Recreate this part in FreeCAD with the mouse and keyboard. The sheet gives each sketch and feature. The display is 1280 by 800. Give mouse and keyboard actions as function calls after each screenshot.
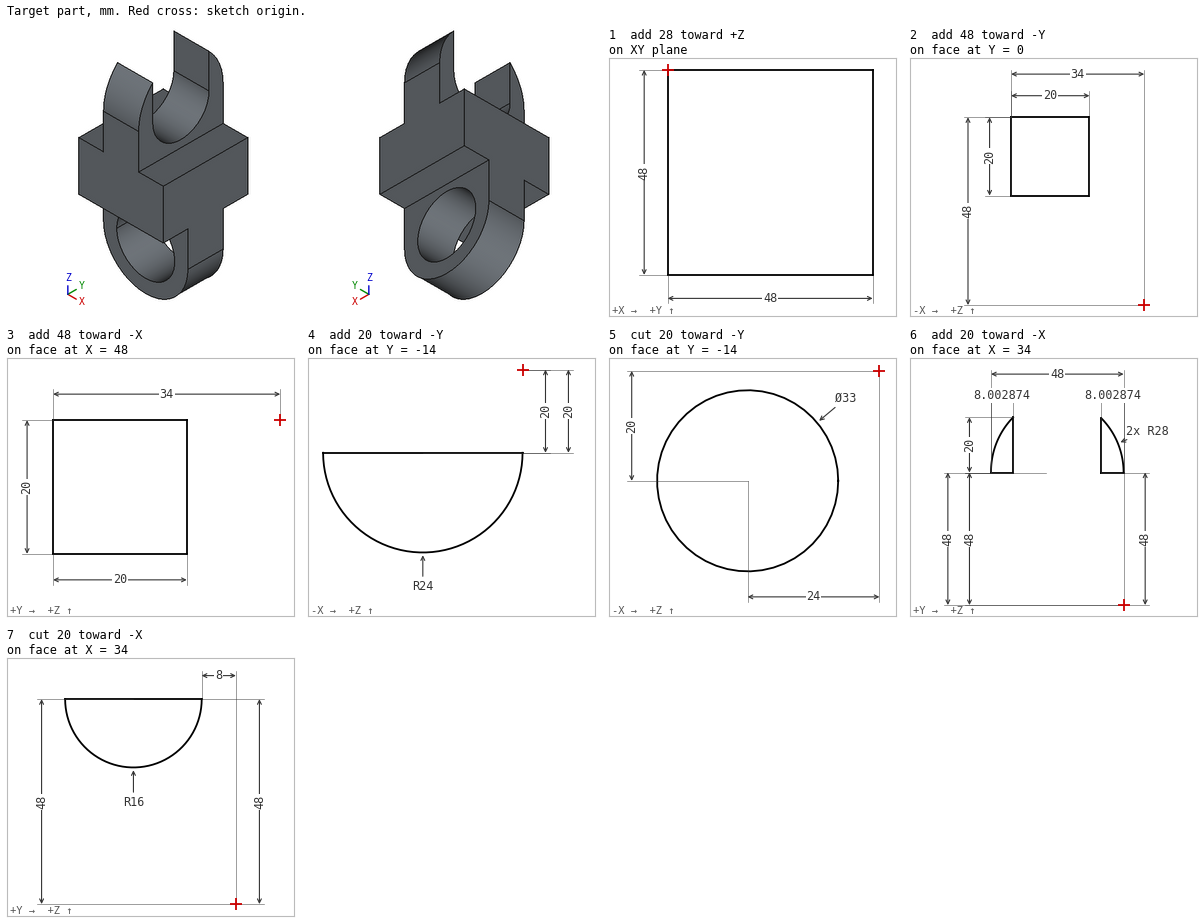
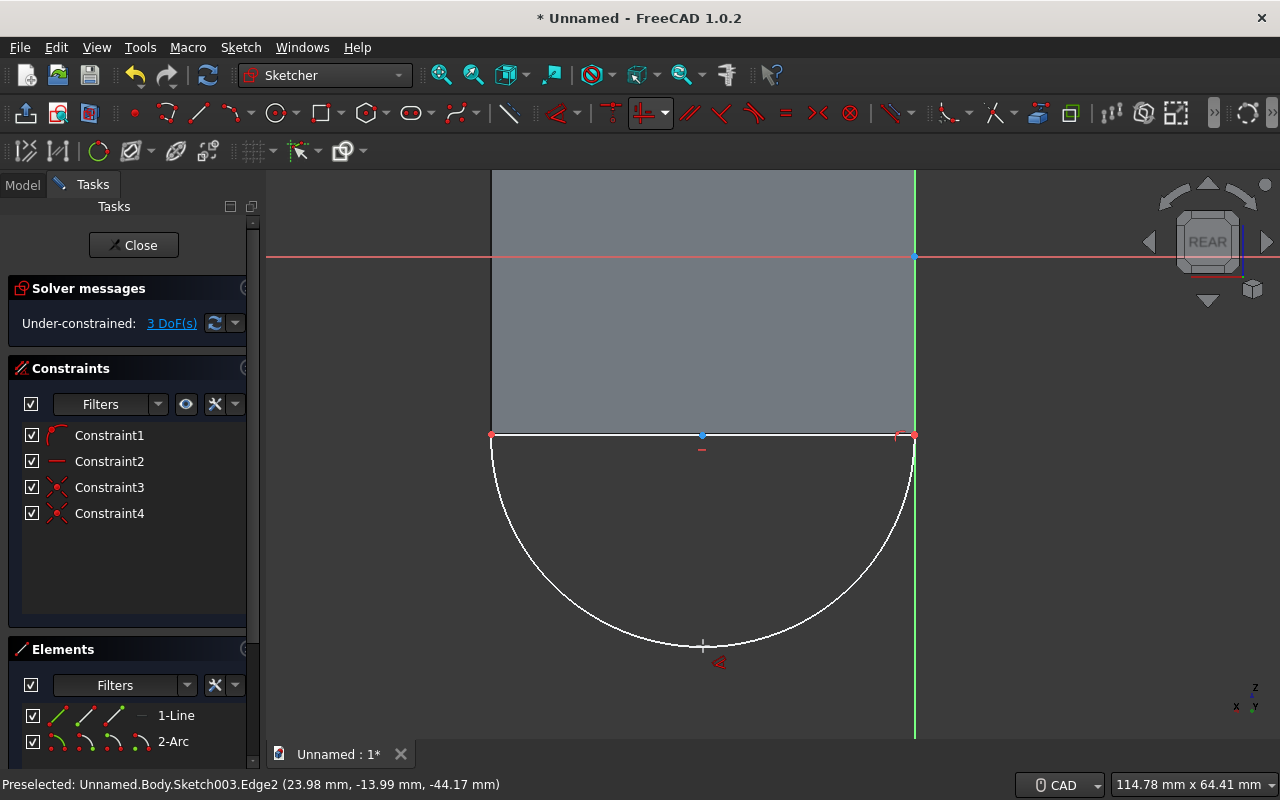
click(578, 607)
click(559, 633)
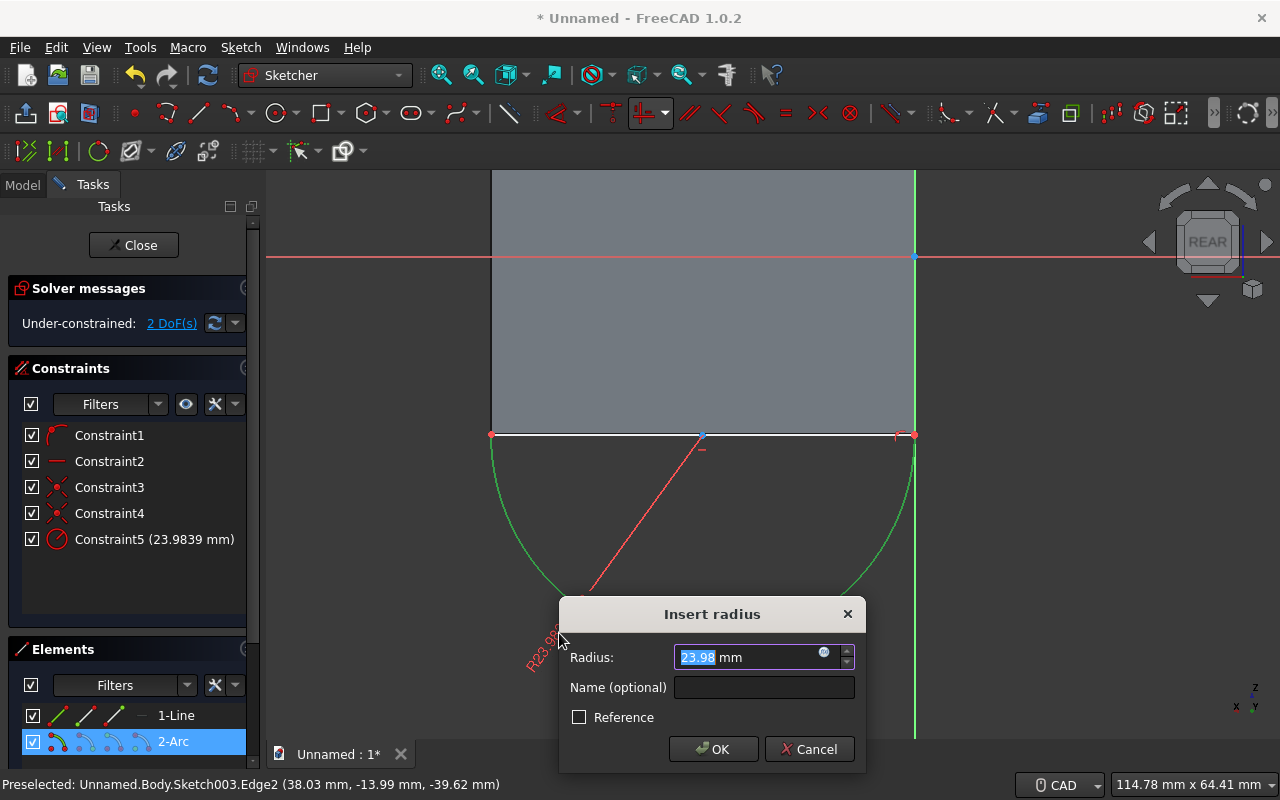
text(24)
key(Return)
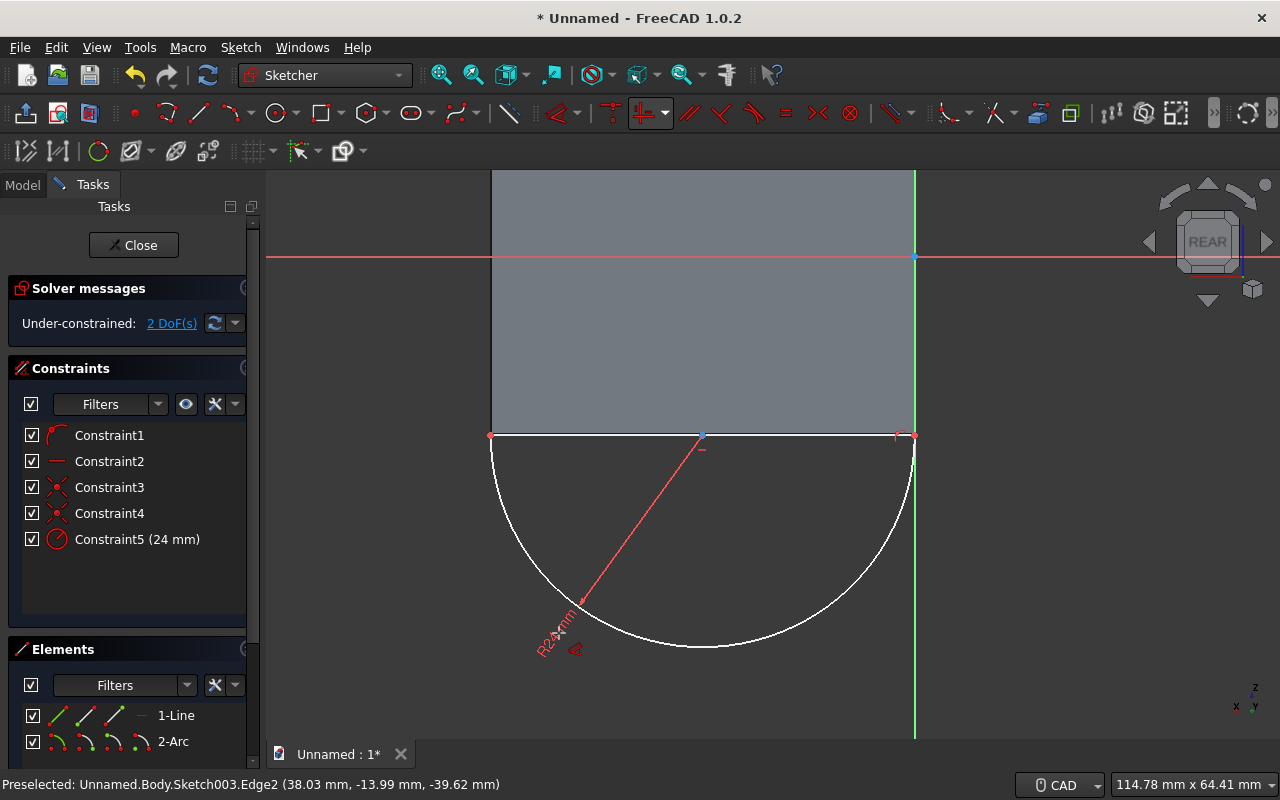
click(915, 435)
click(949, 346)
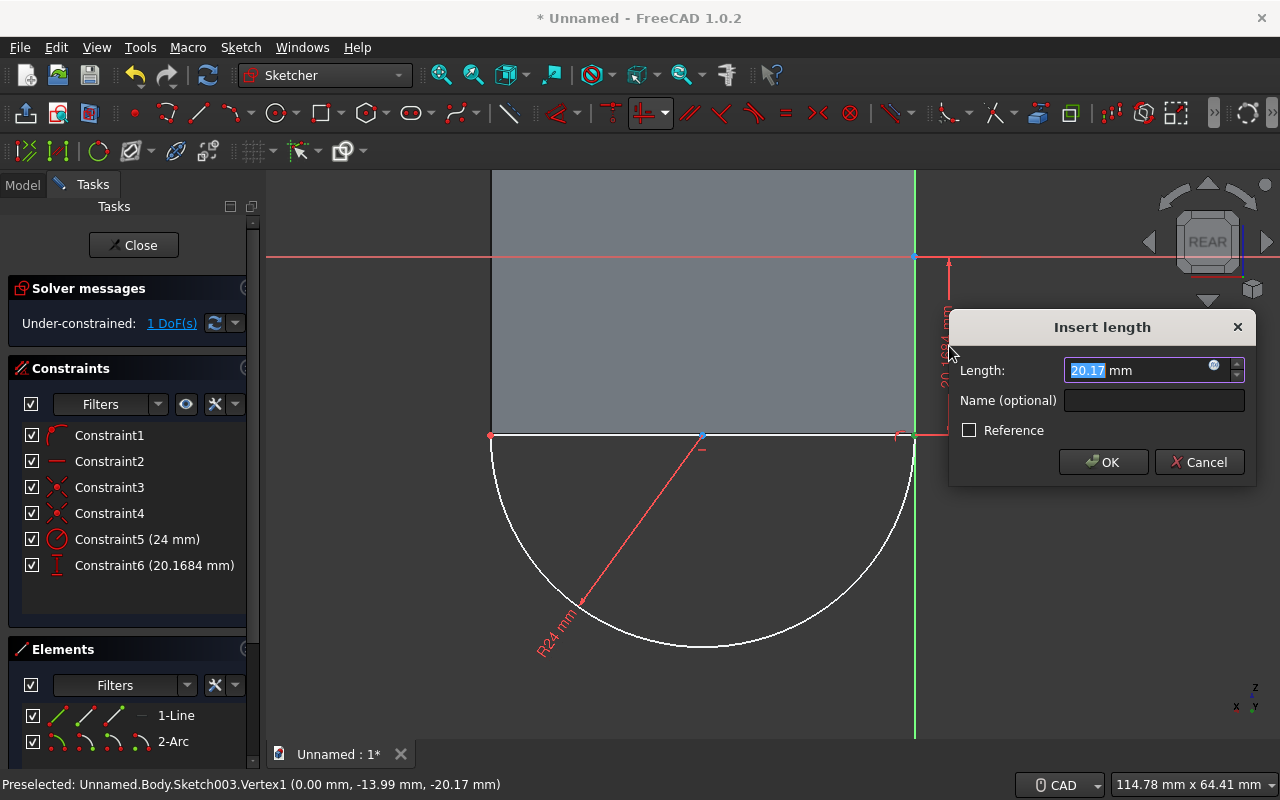
text(20)
key(Return)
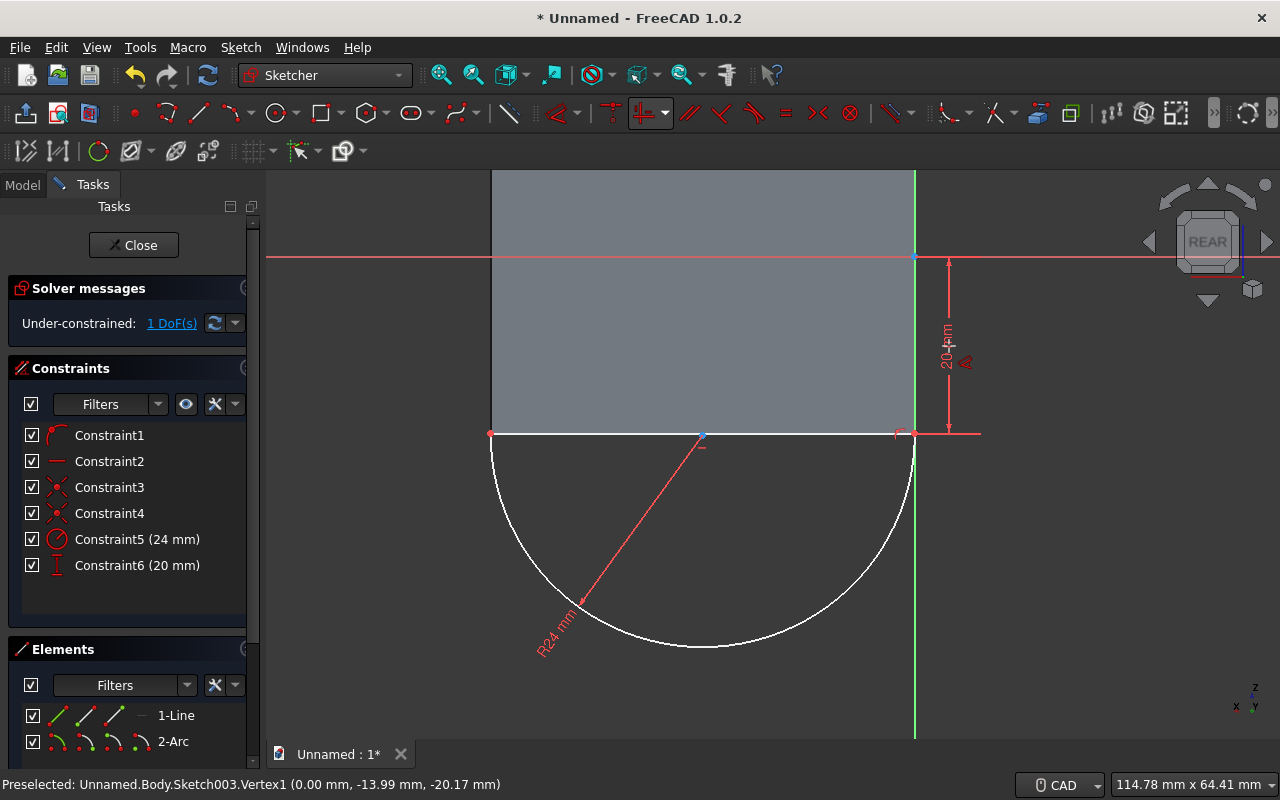
click(703, 435)
click(949, 305)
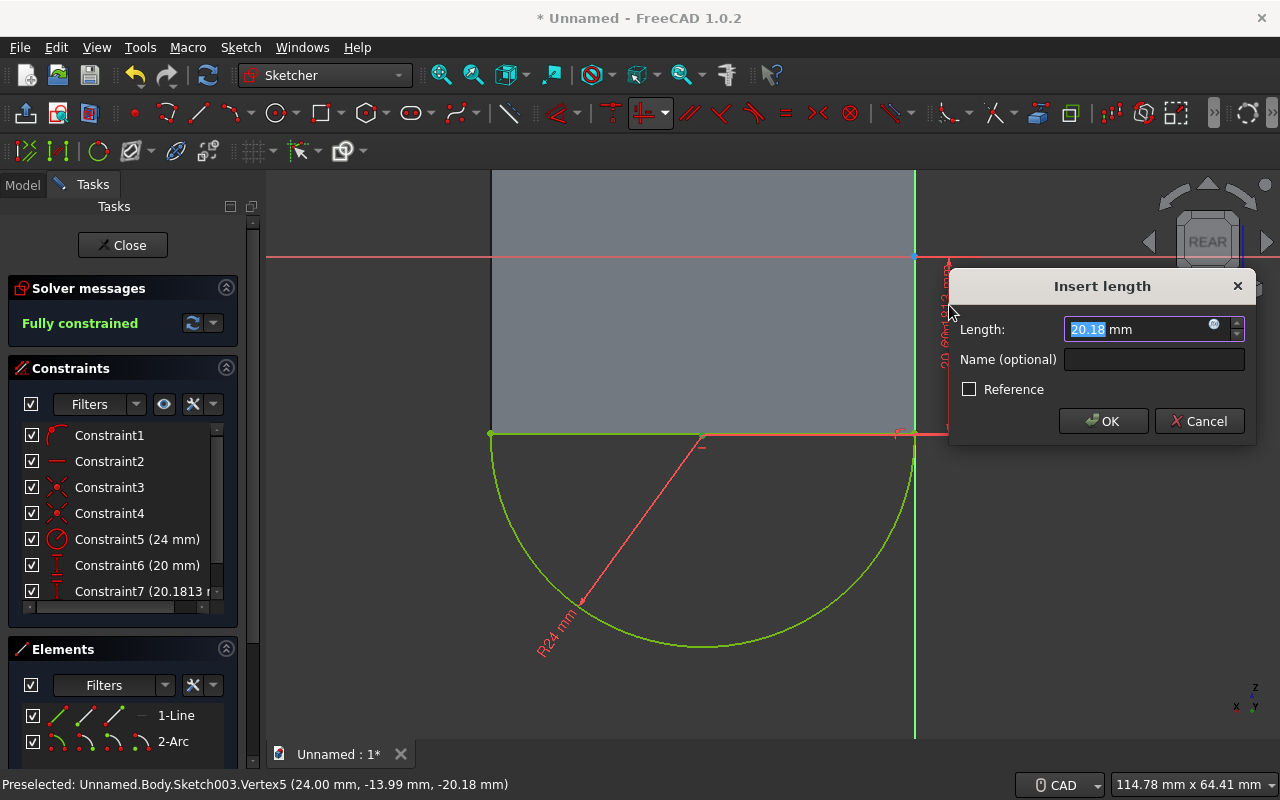
text(20)
key(Return)
key(Escape)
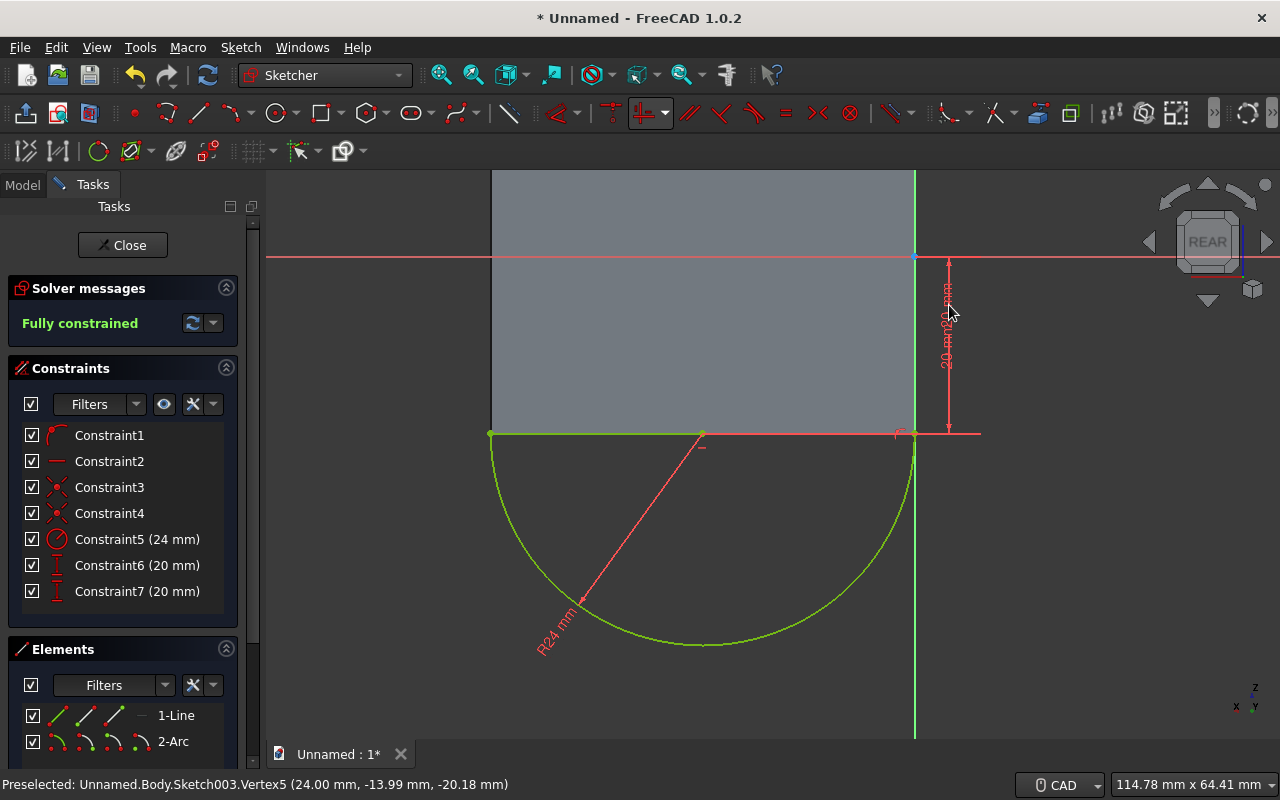
click(123, 245)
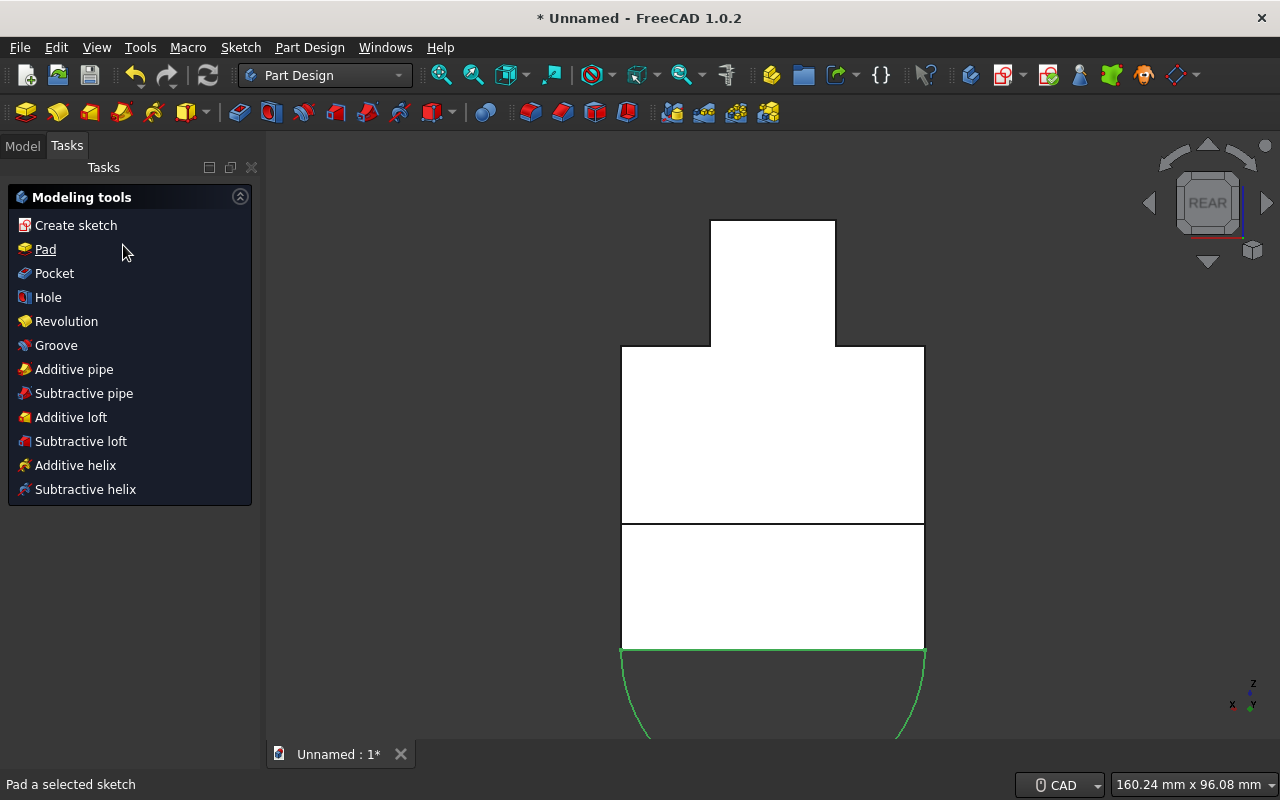
click(26, 112)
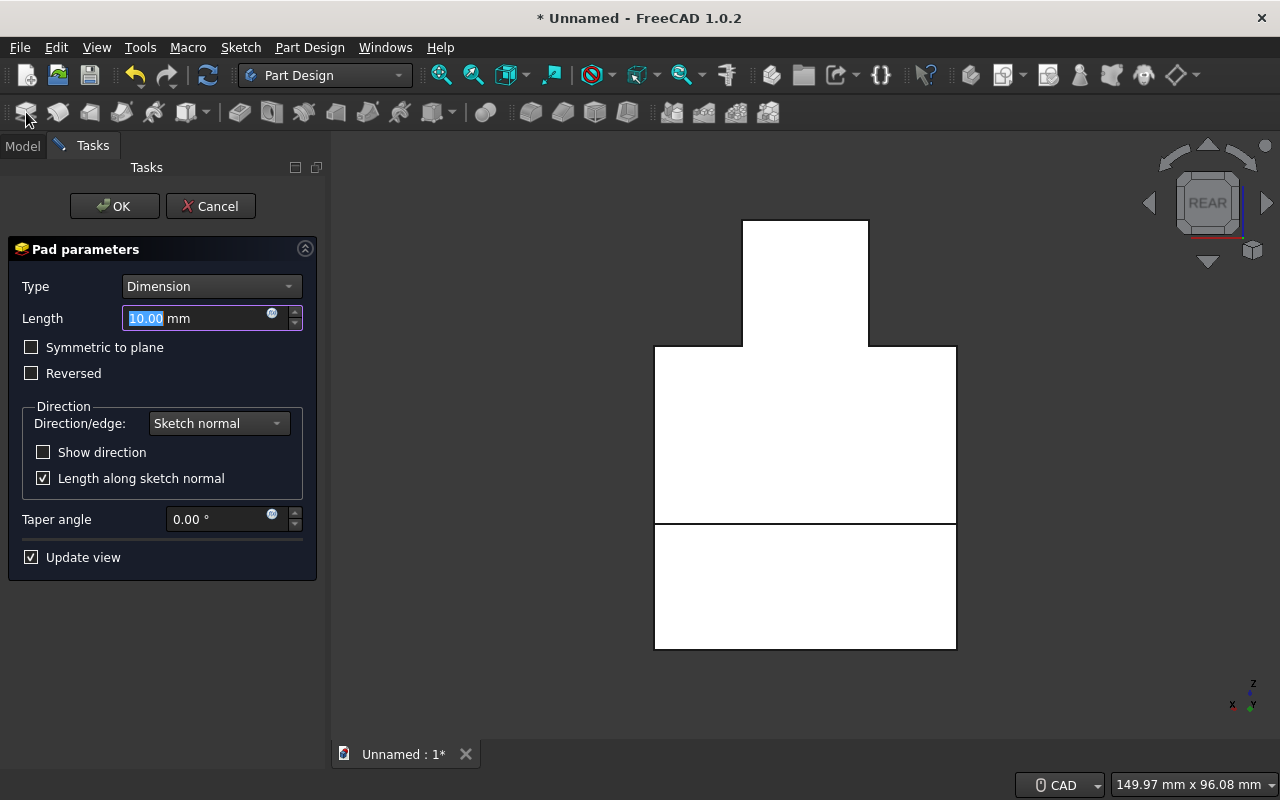
text(20)
key(Tab)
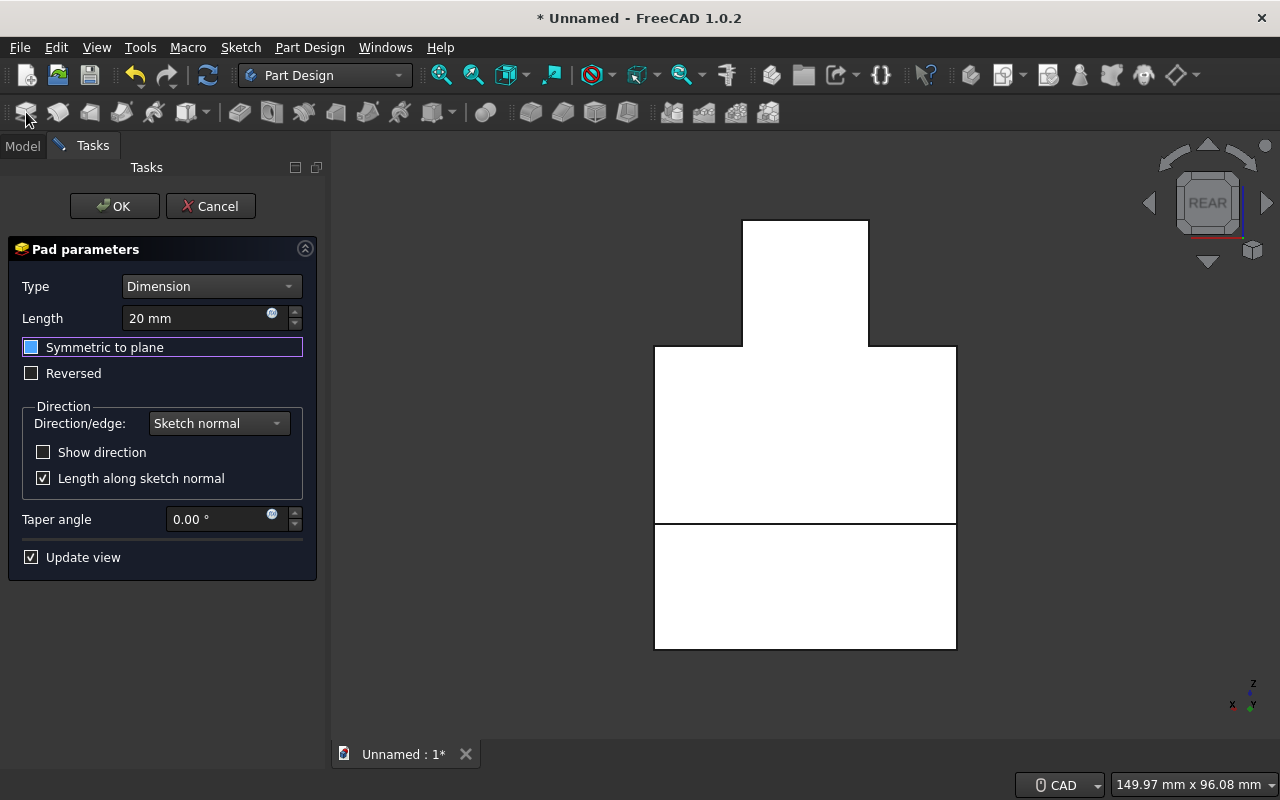
click(30, 373)